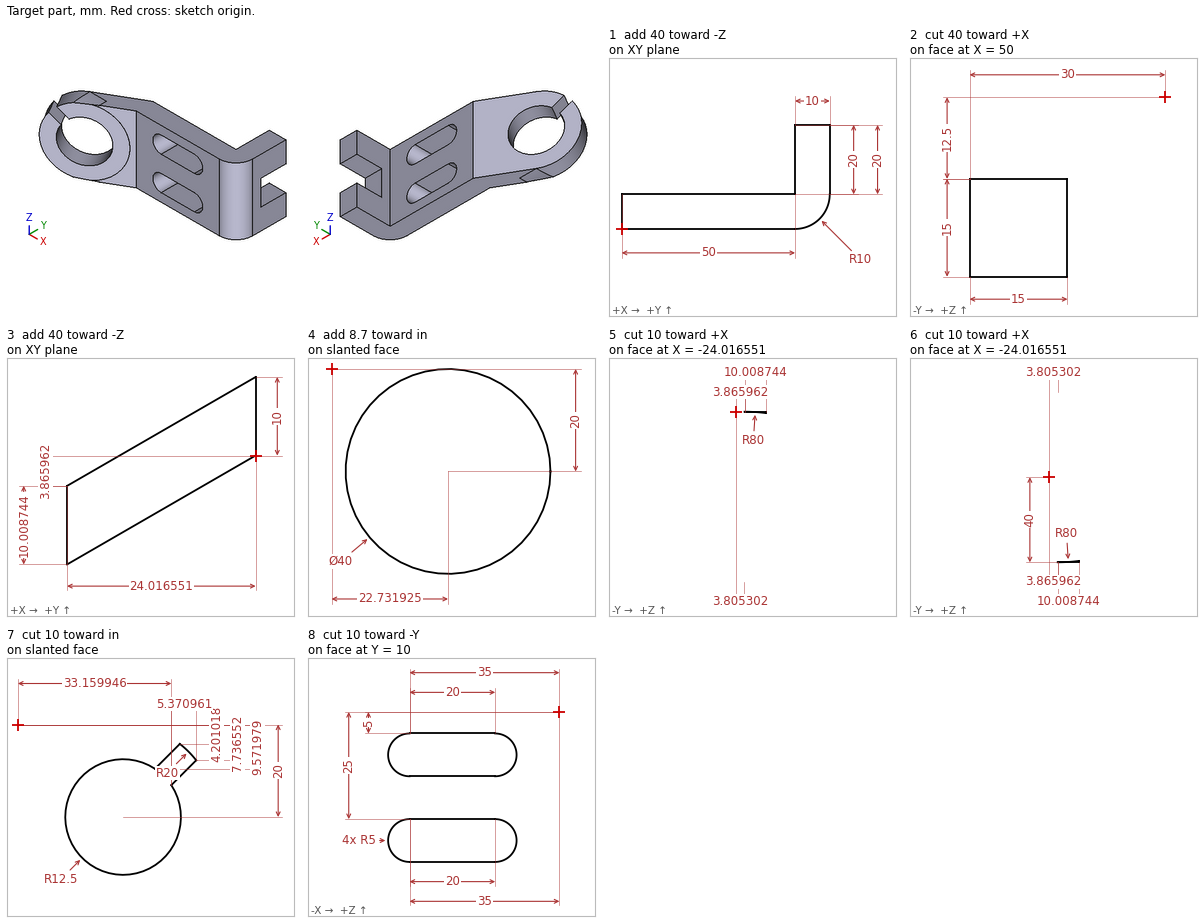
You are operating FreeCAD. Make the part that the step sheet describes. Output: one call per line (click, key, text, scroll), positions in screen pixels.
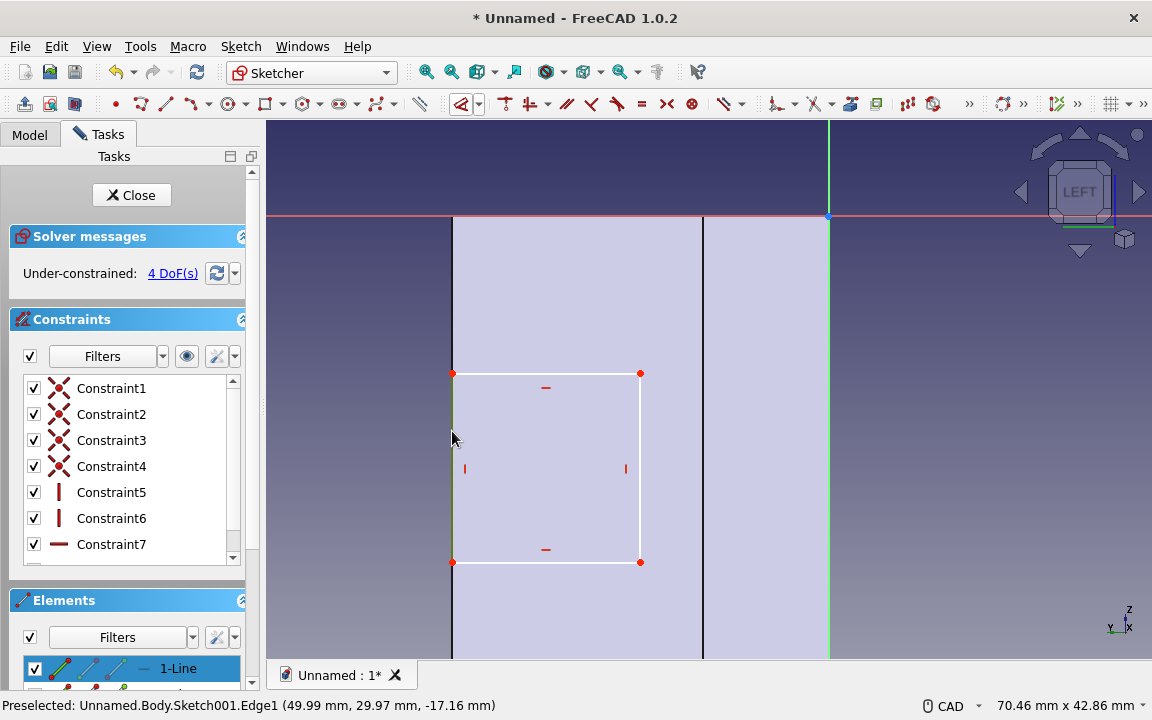
key(i)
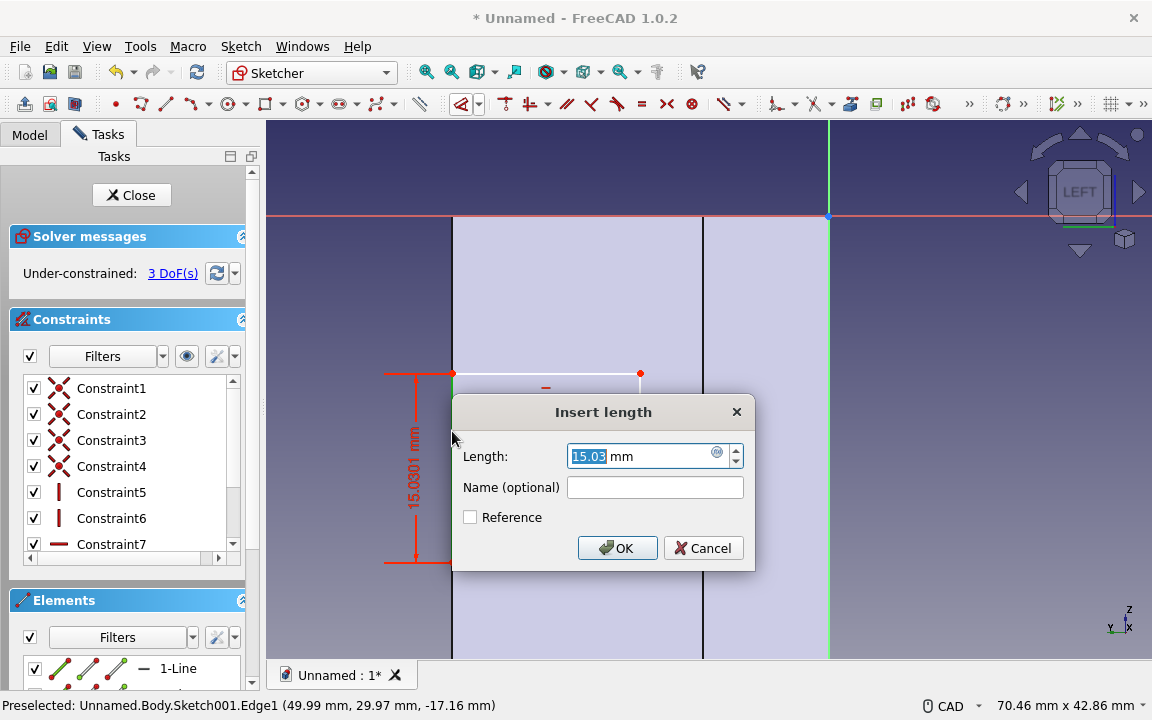
text(15)
key(Return)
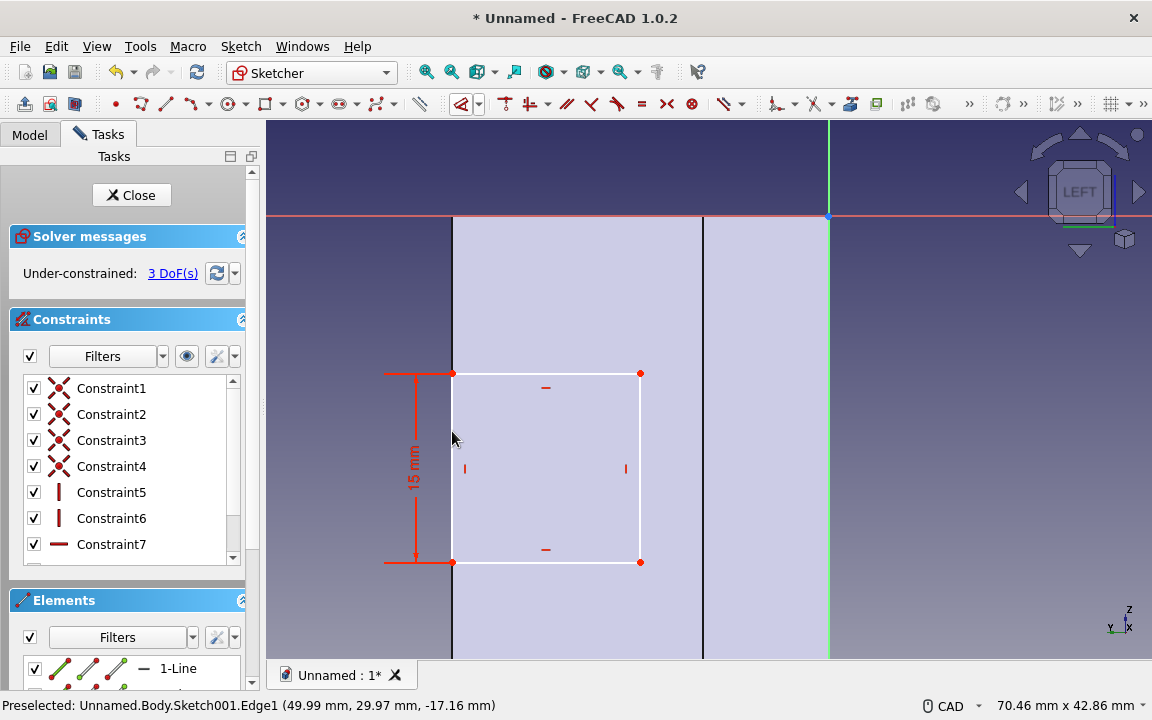
click(508, 563)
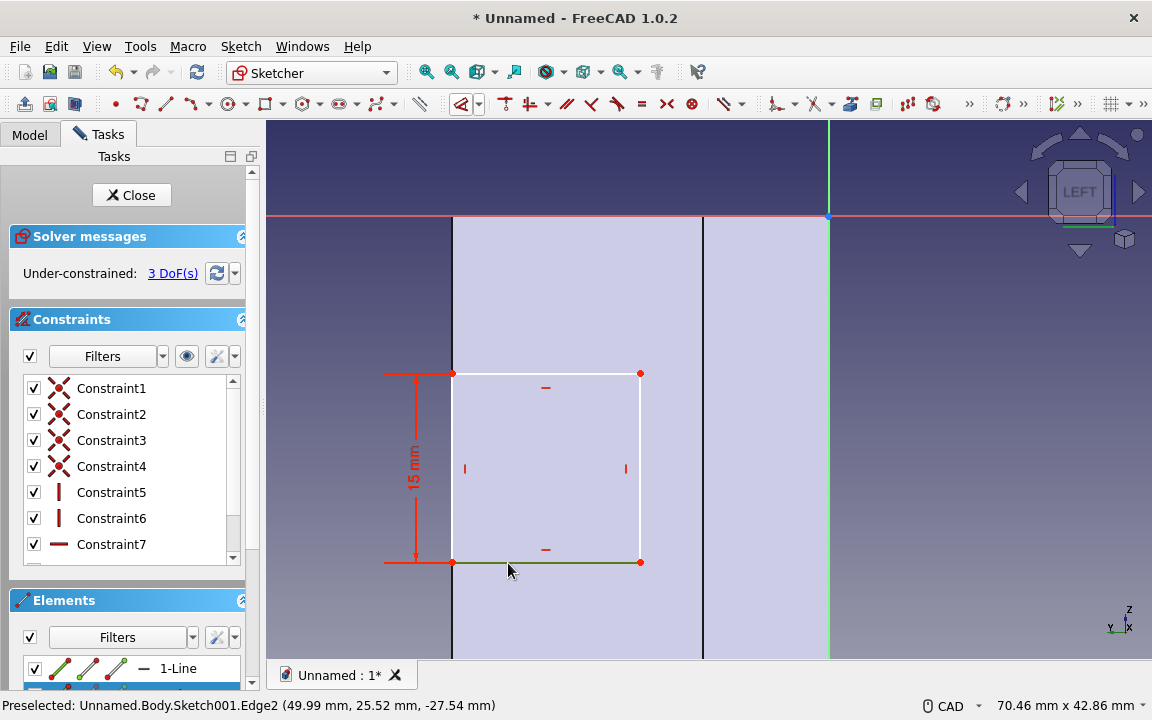
click(478, 104)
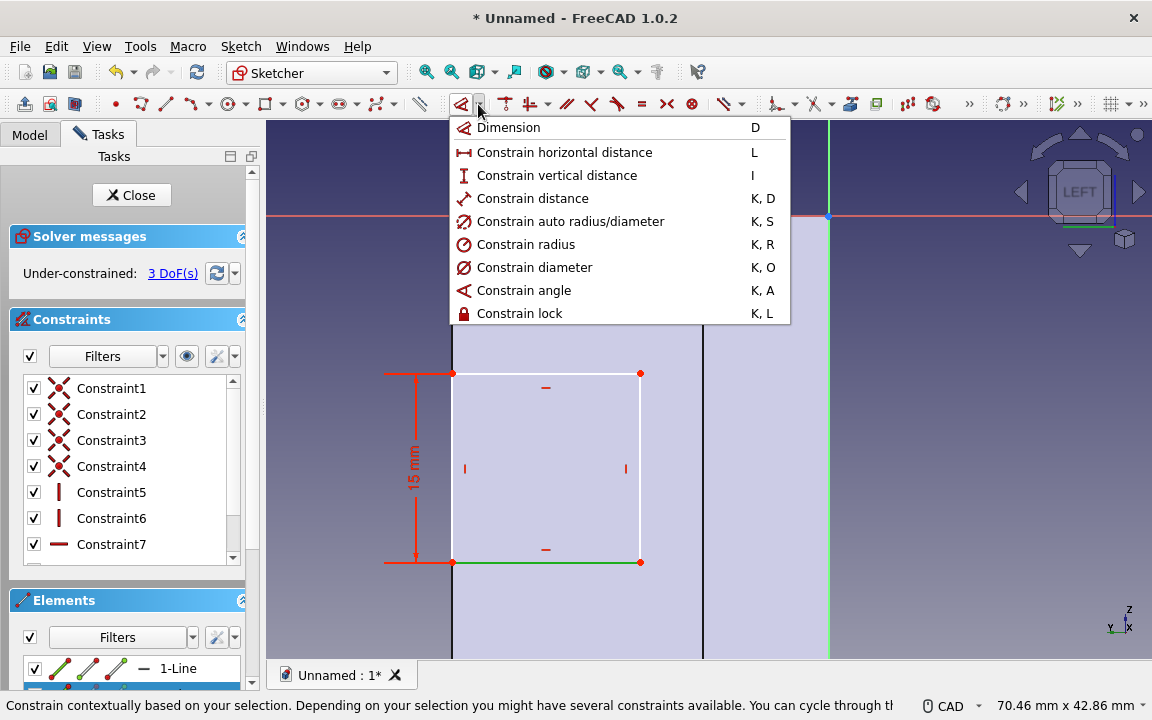
click(620, 152)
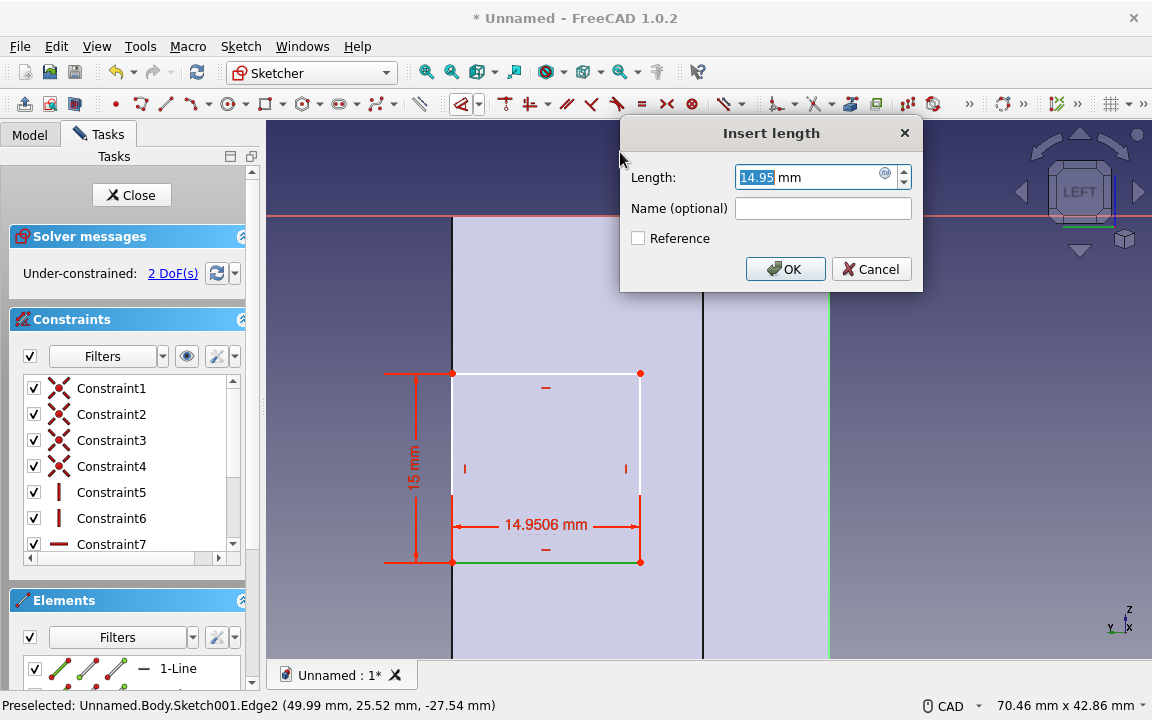
text(15)
key(Return)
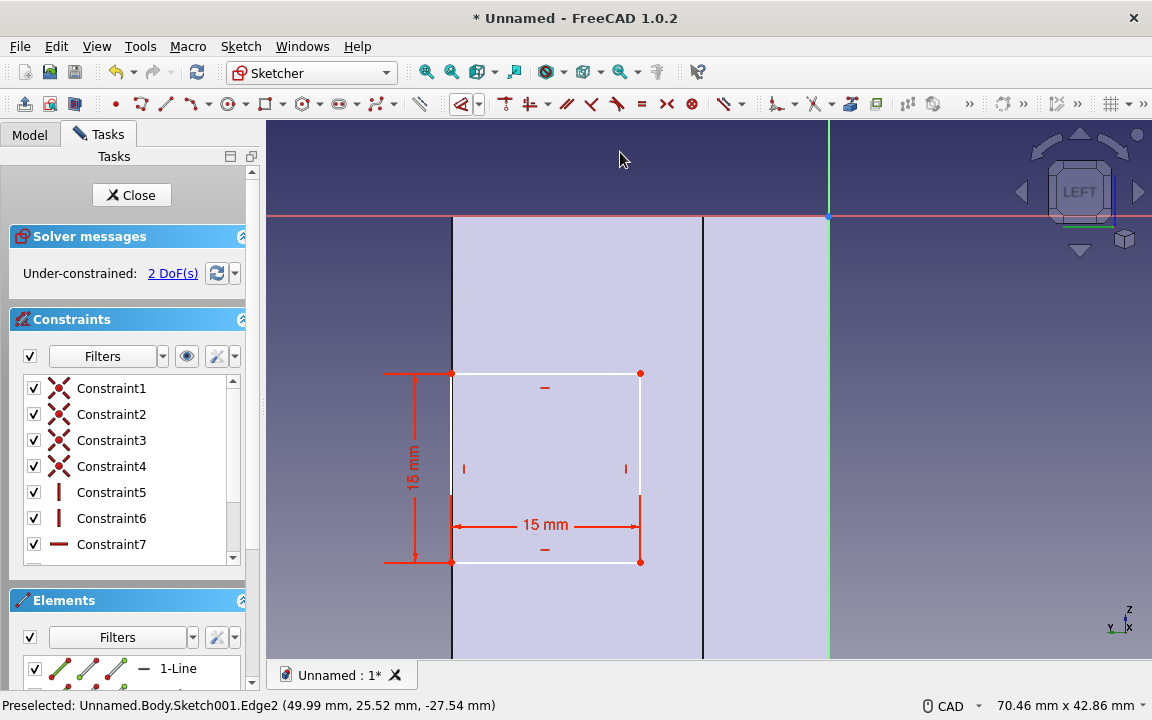
click(451, 374)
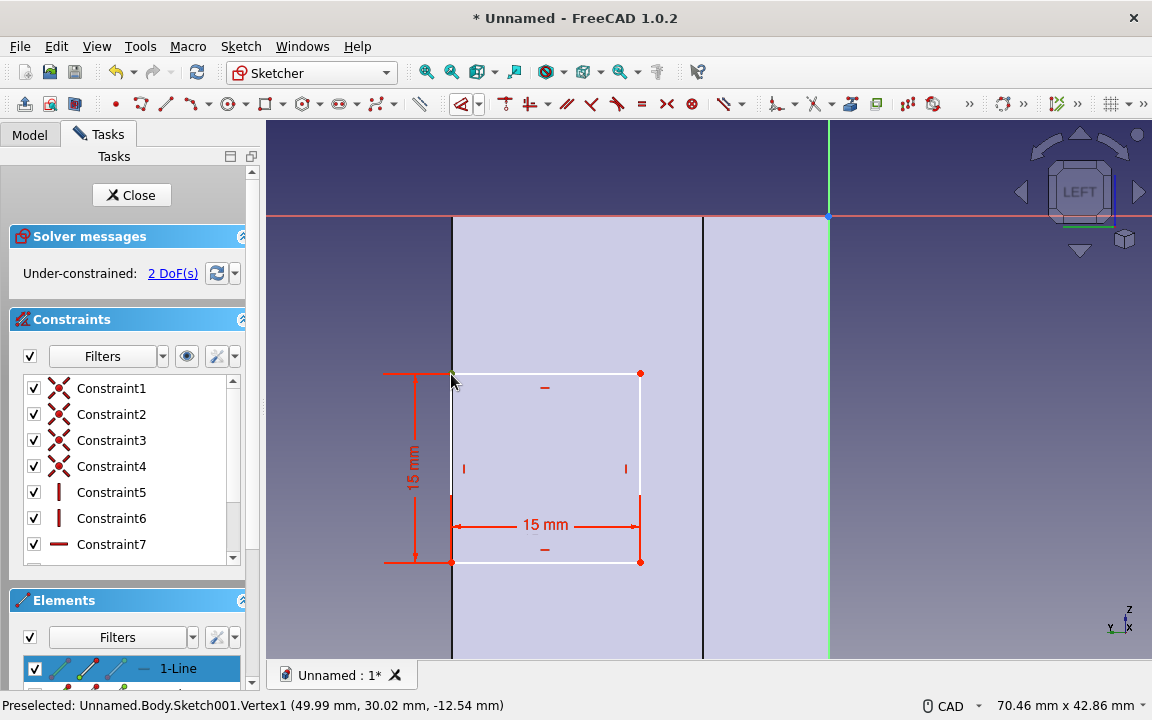
key(l)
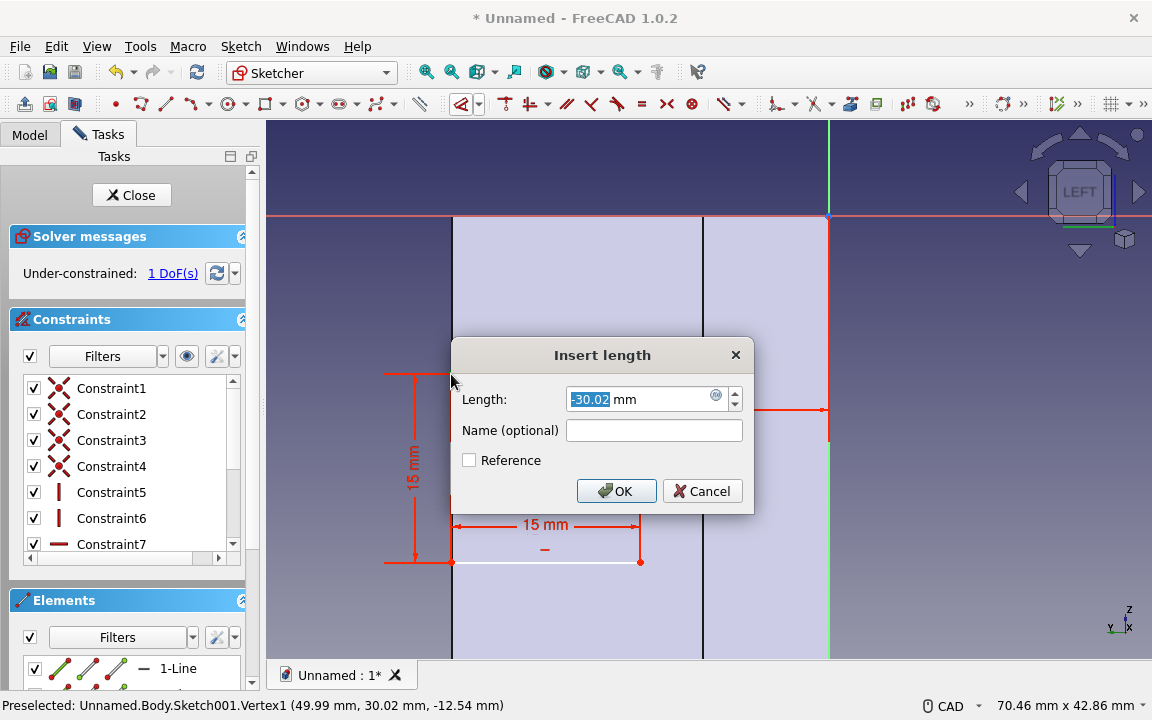
text(-30)
key(Return)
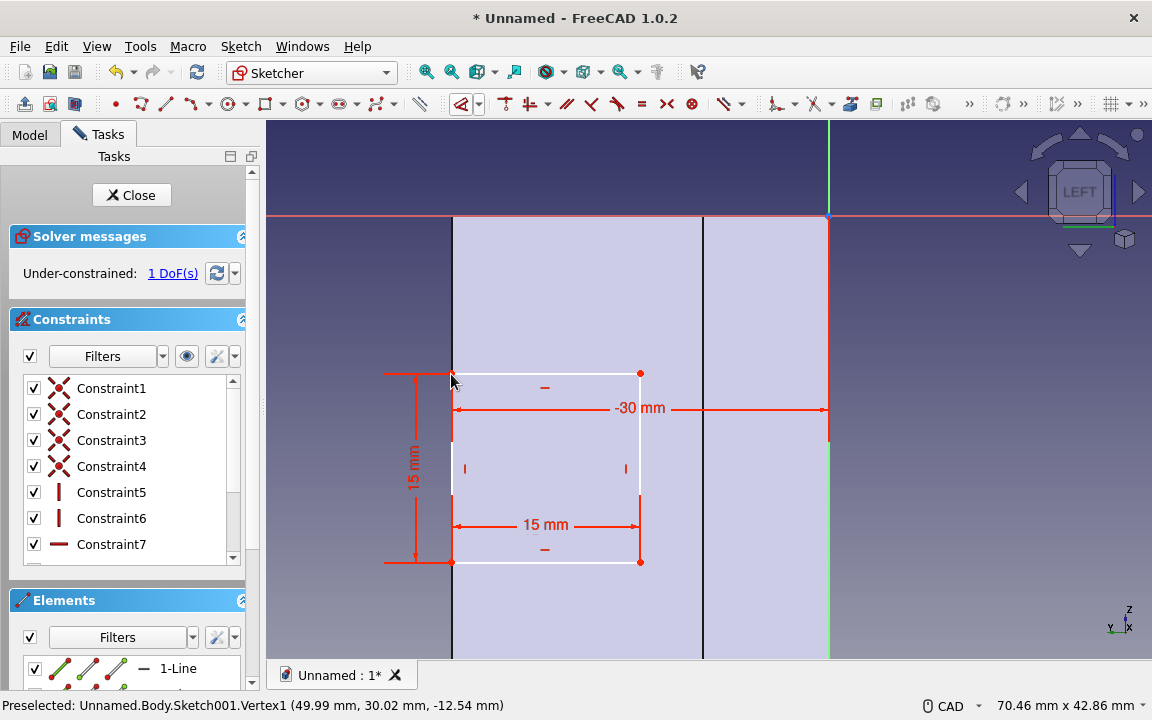
click(452, 374)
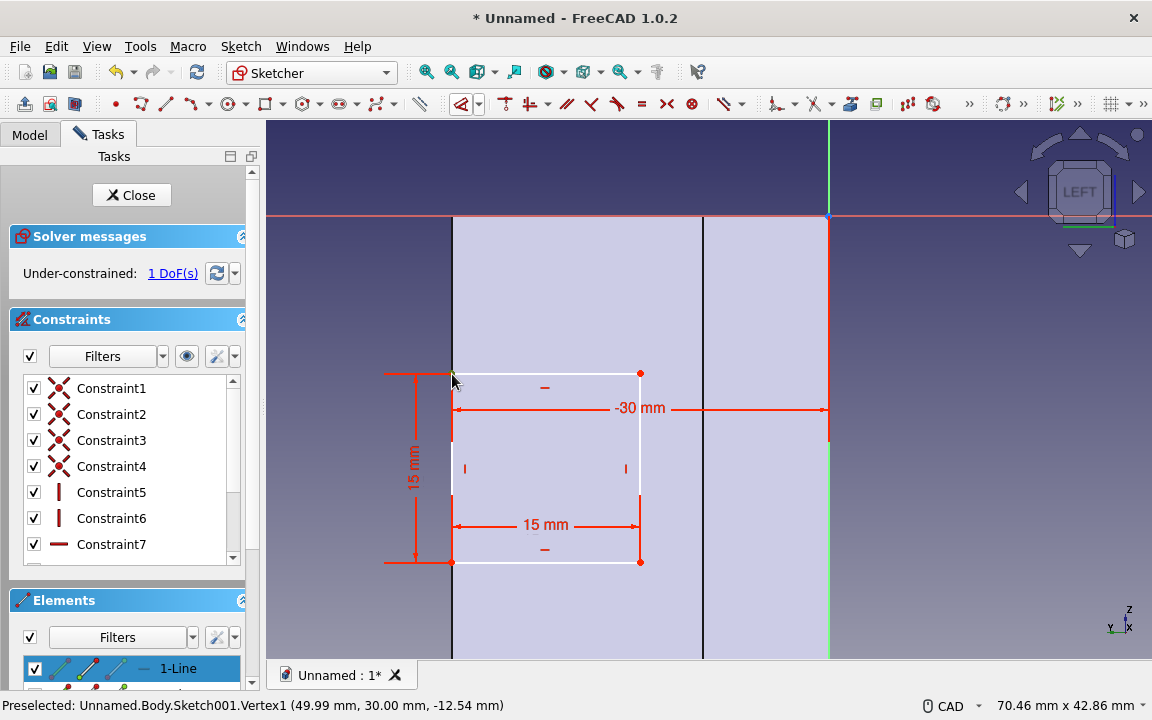
key(i)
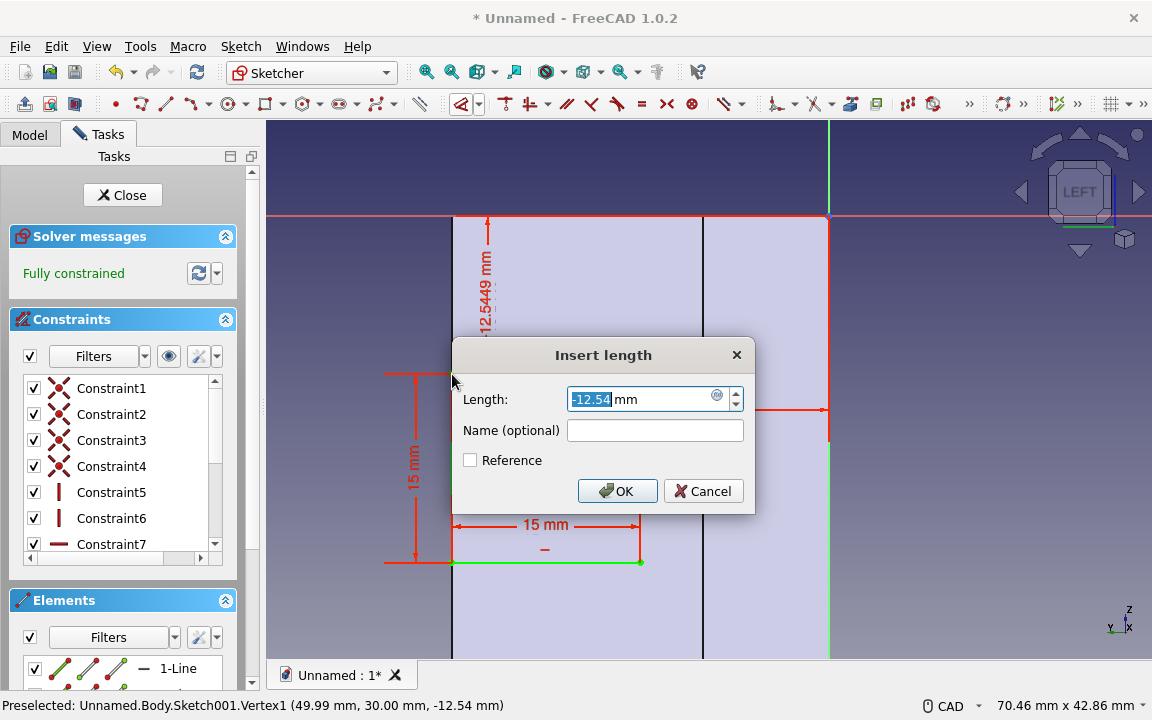
text(-12.5)
key(Return)